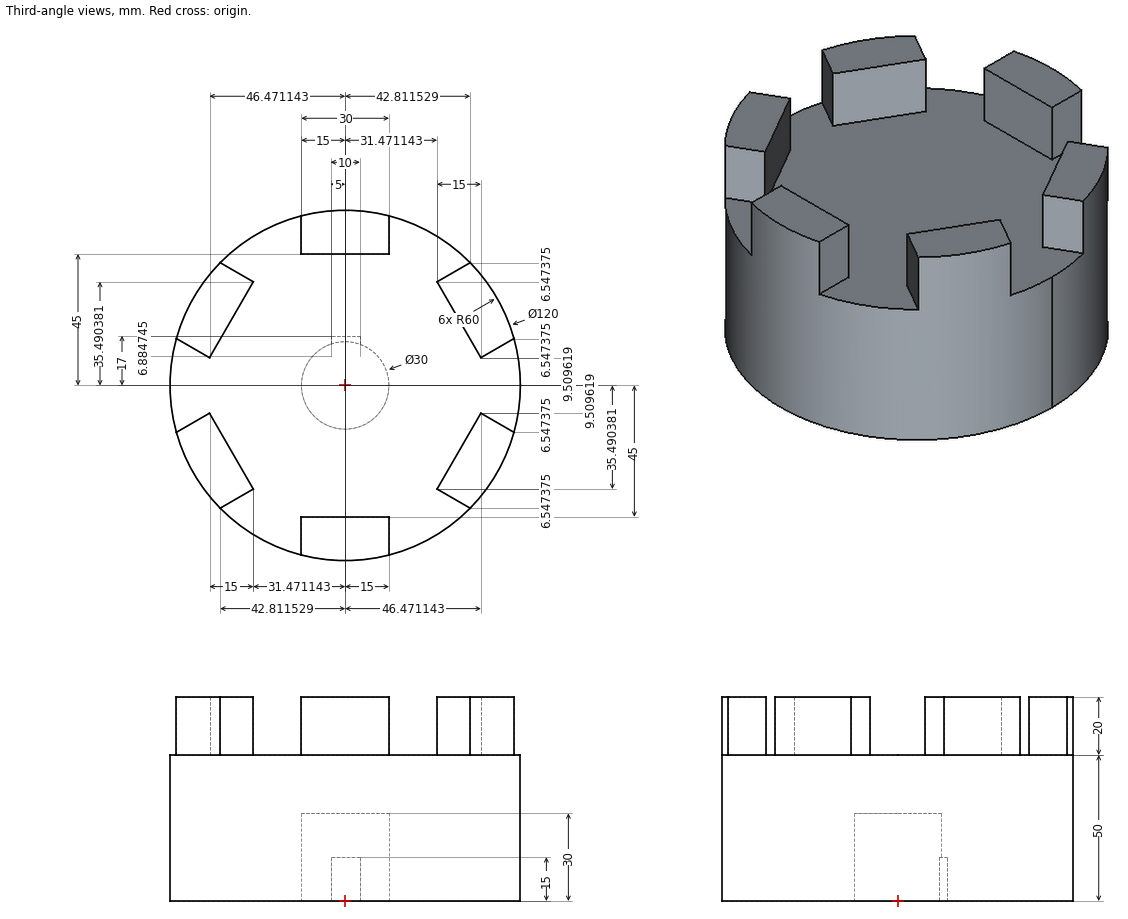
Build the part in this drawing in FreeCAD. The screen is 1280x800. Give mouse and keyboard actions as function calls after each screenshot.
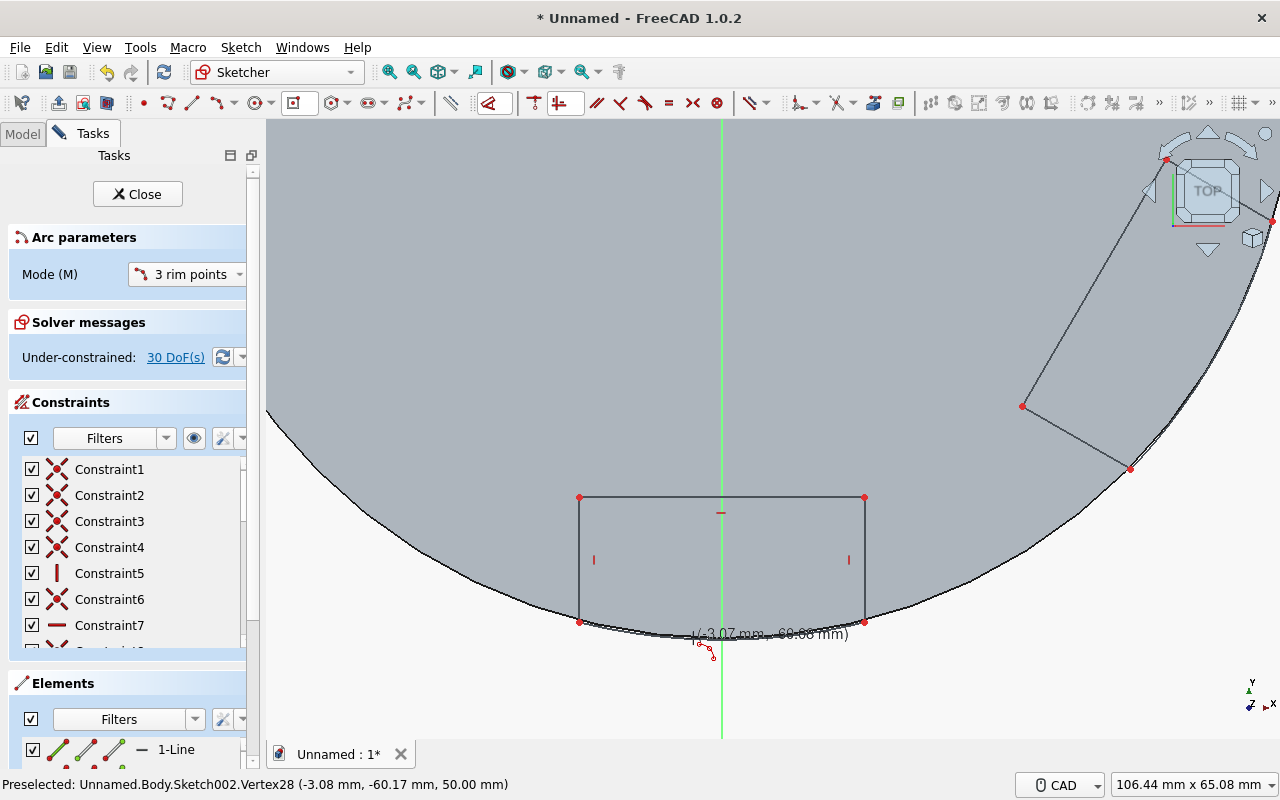
key(g)
key(m)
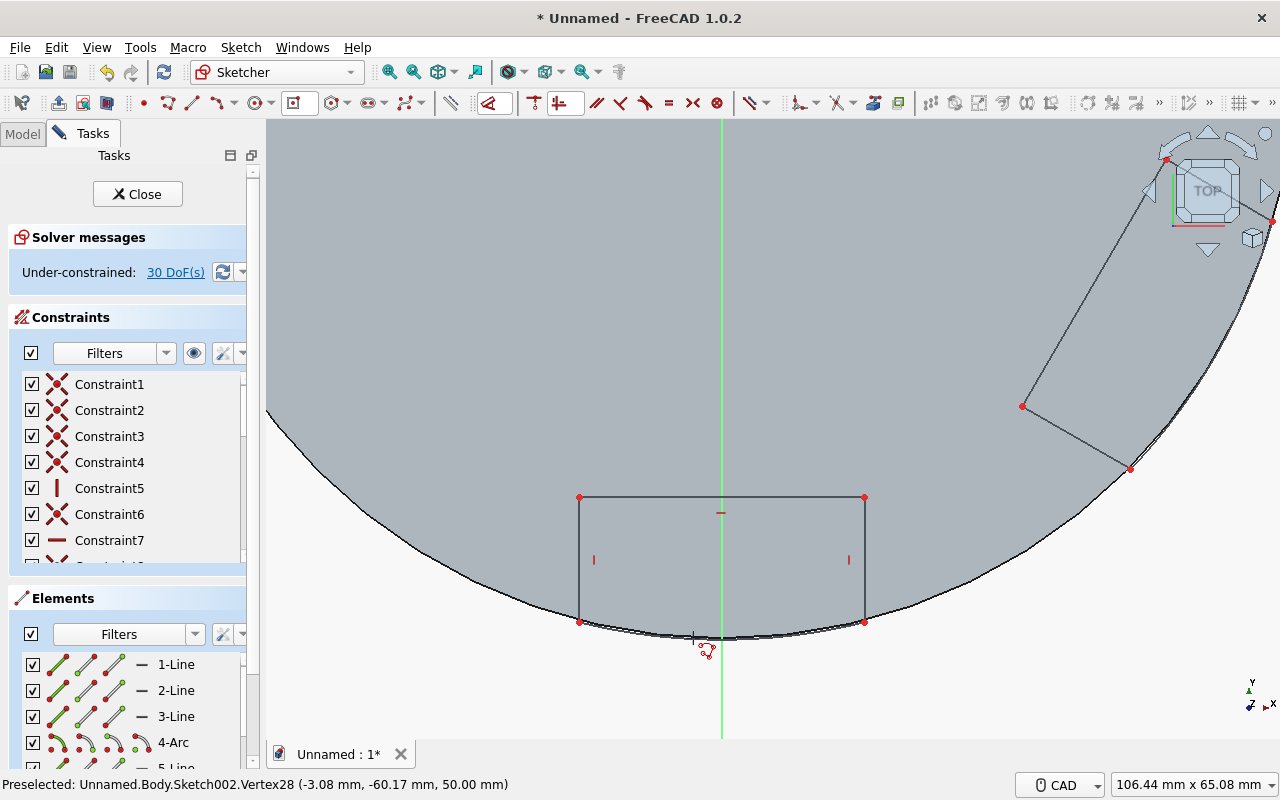
click(314, 467)
click(422, 405)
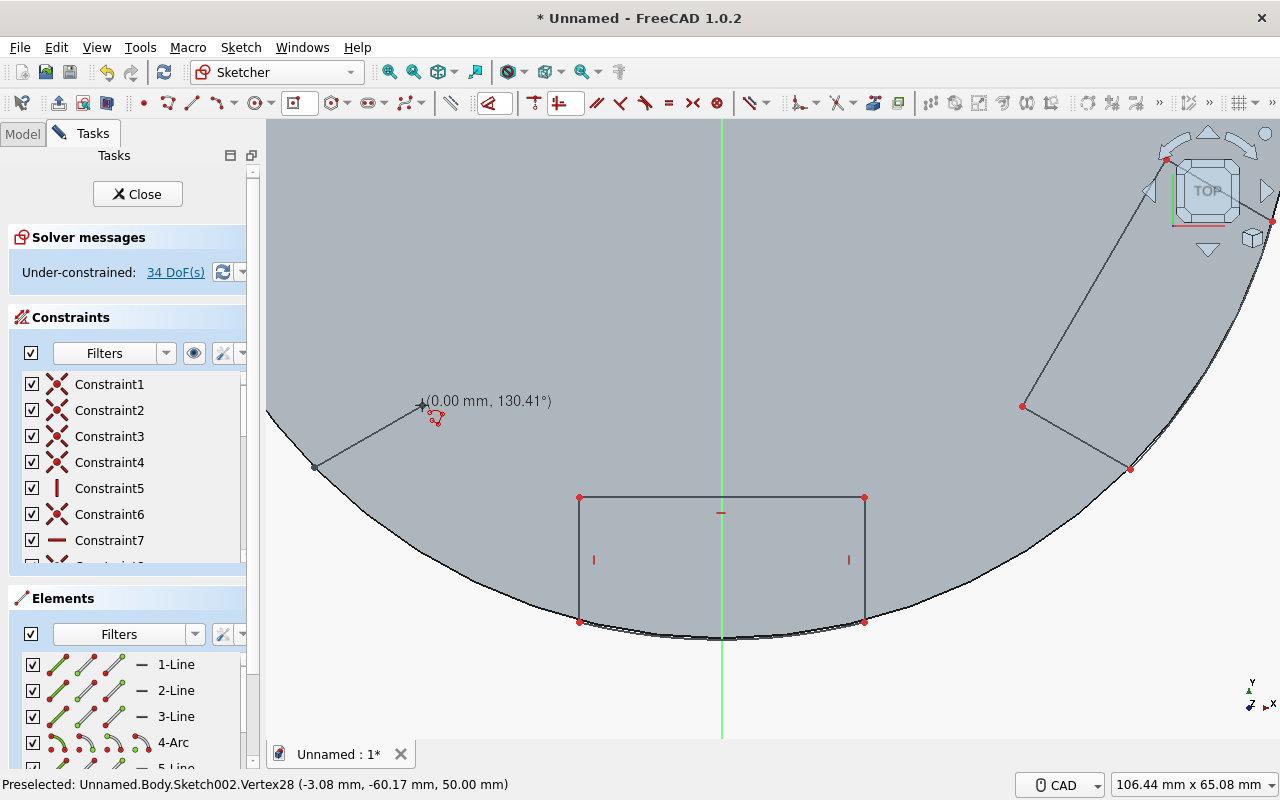
scroll(694, 640, down, 5)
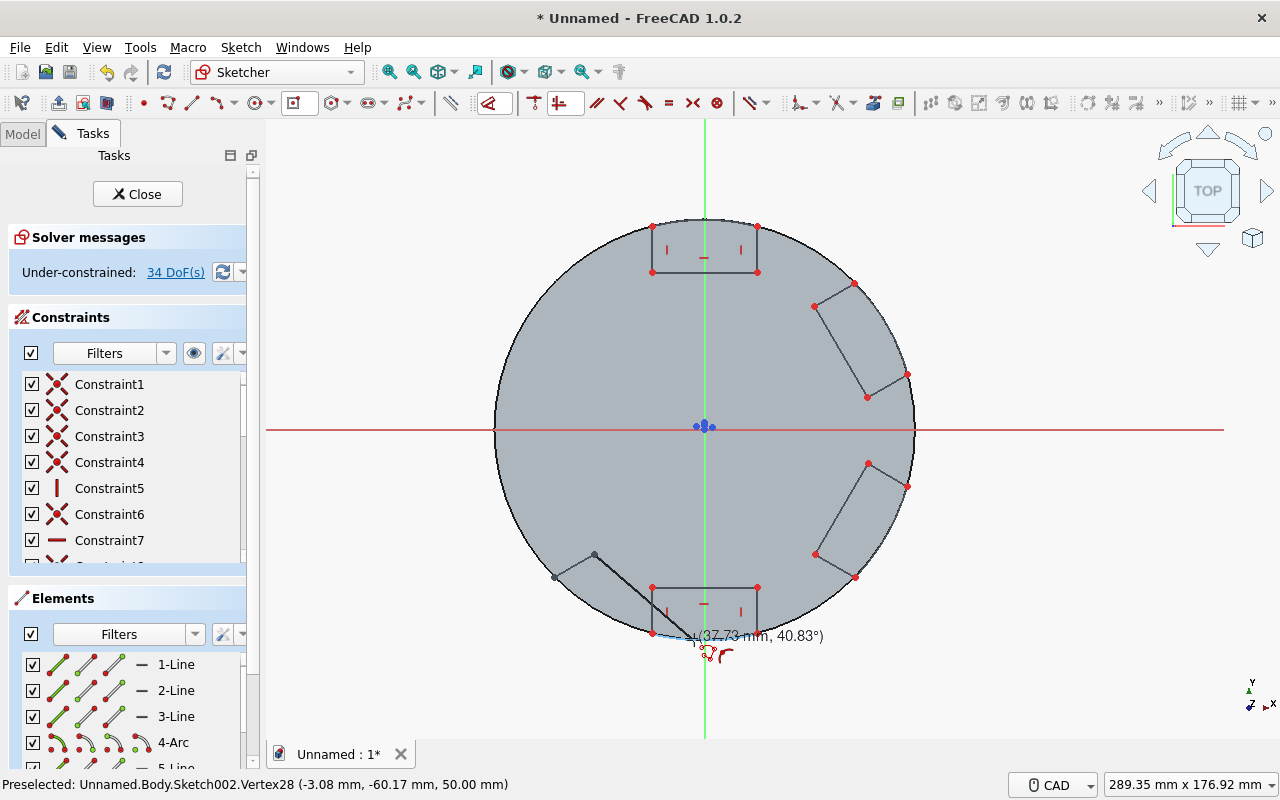
click(542, 463)
click(502, 486)
right_click(502, 486)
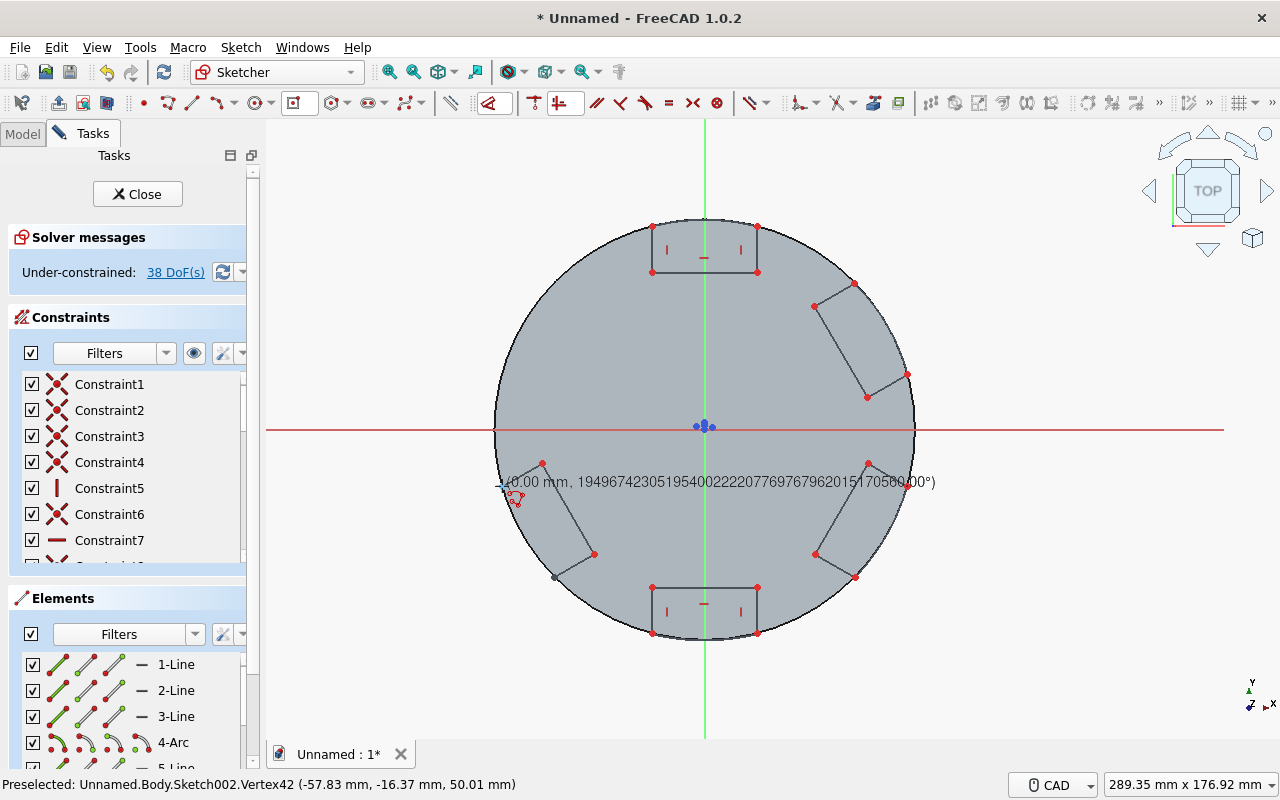
click(218, 104)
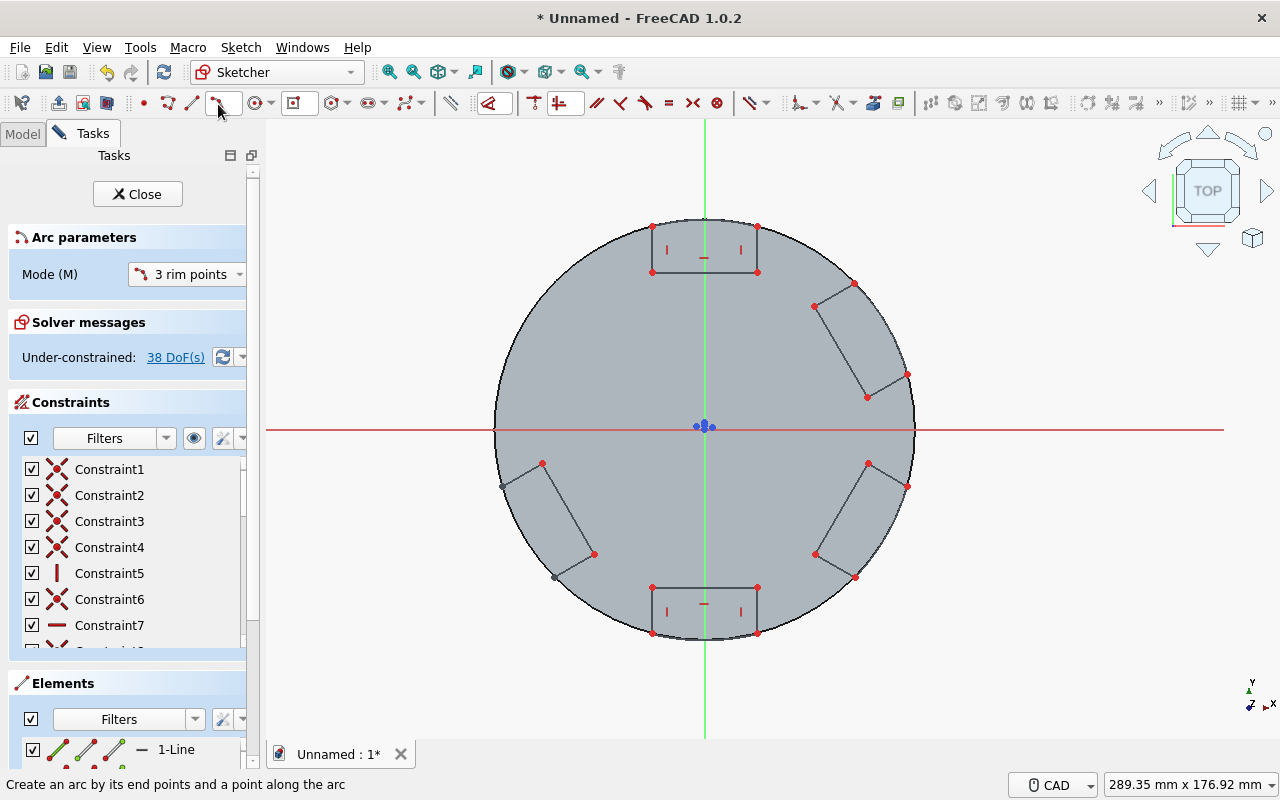
click(502, 487)
click(554, 577)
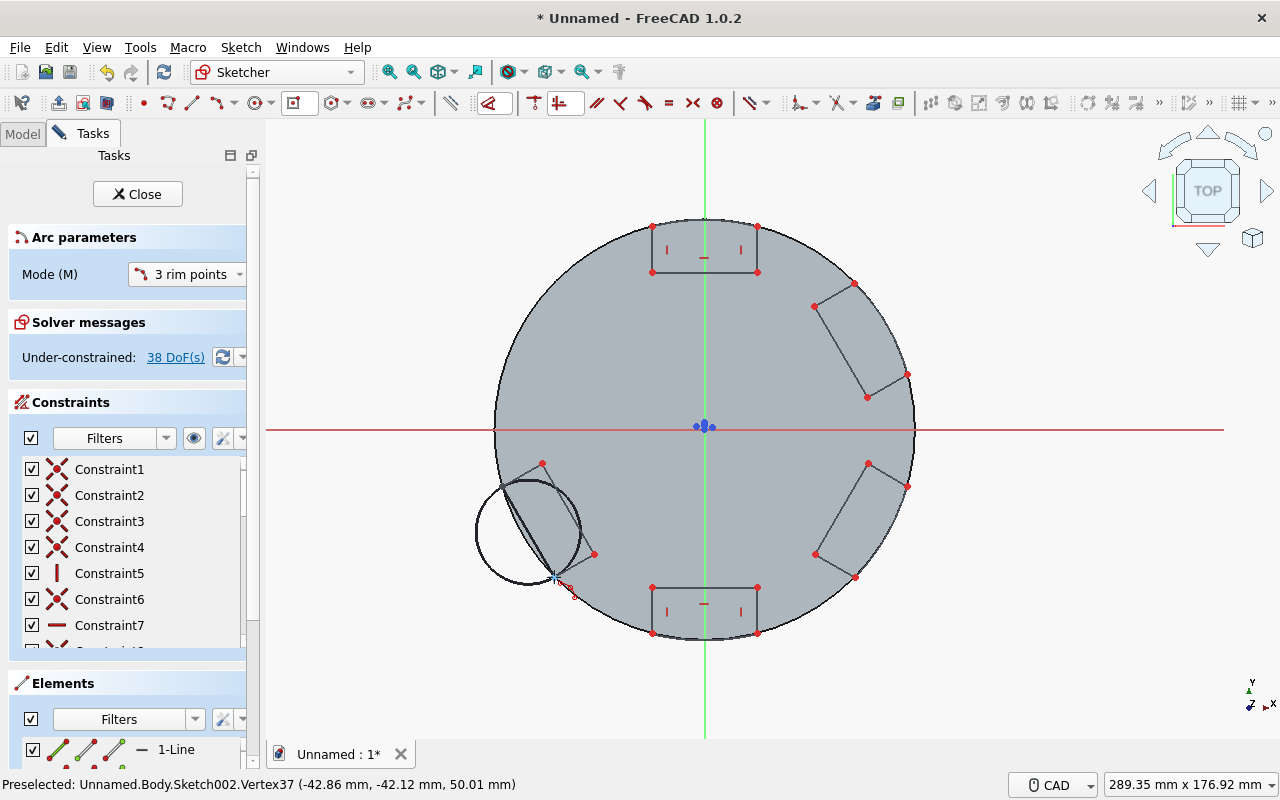
scroll(523, 535, up, 5)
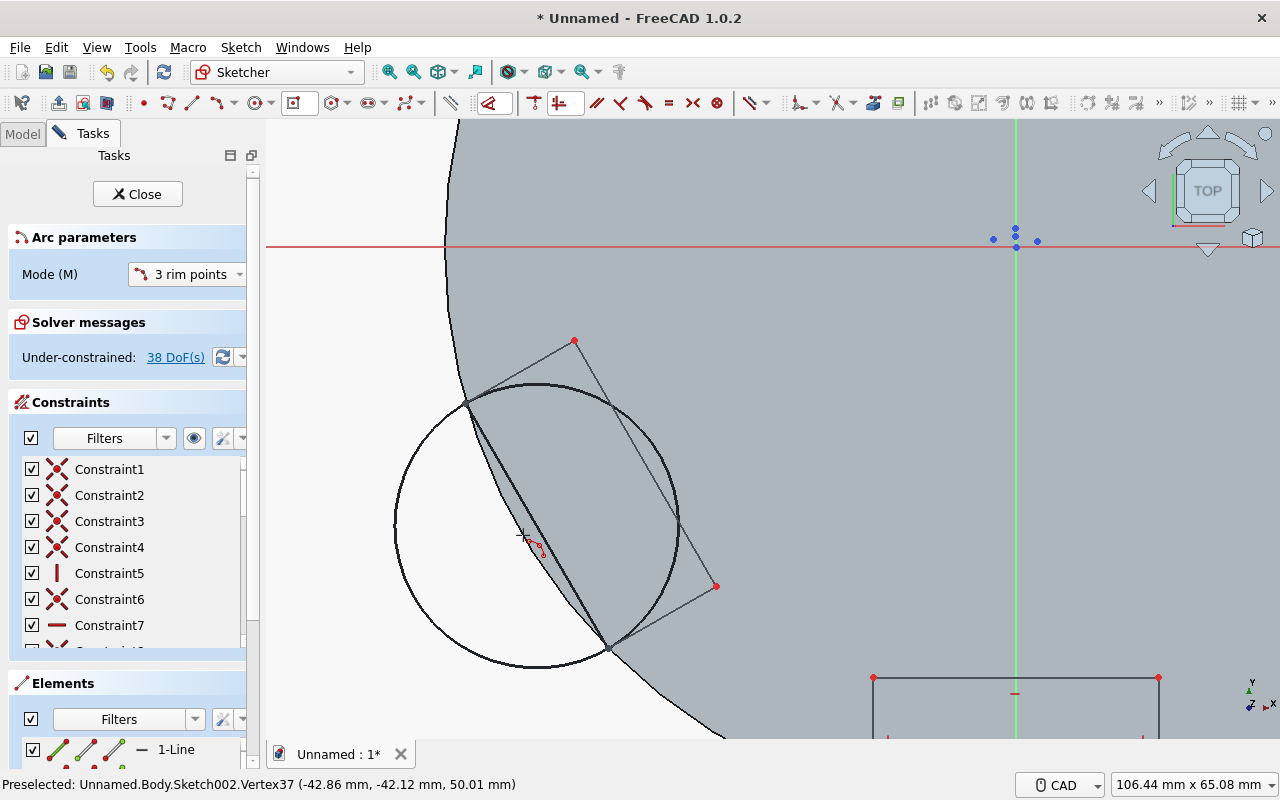
click(521, 533)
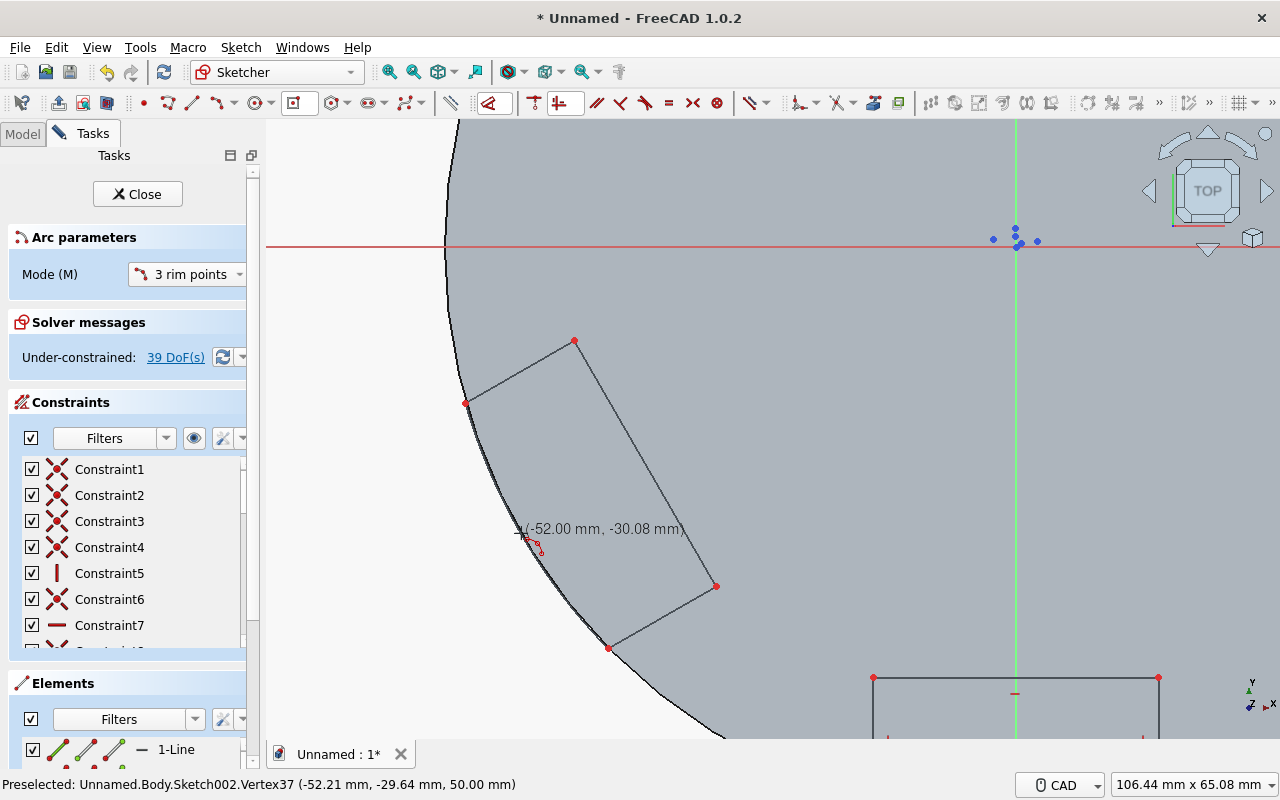
key(g)
key(m)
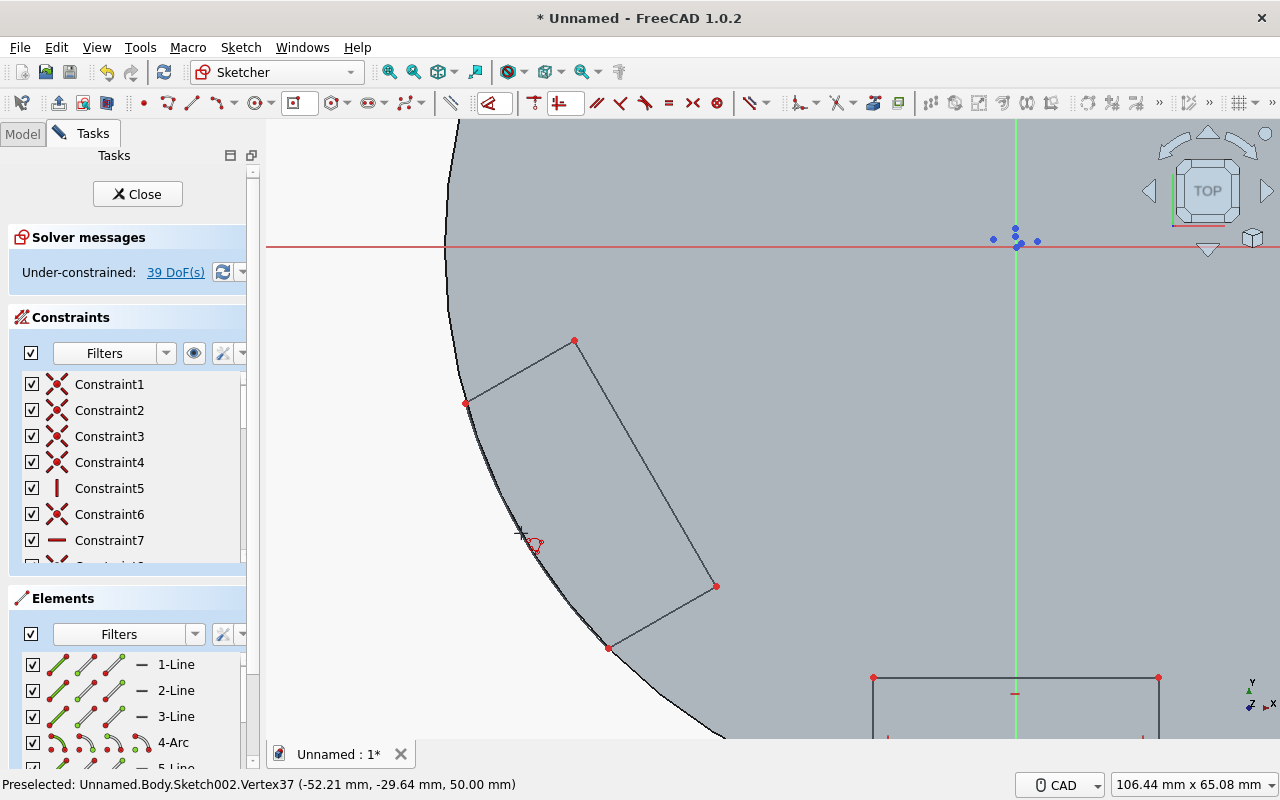
scroll(523, 535, down, 5)